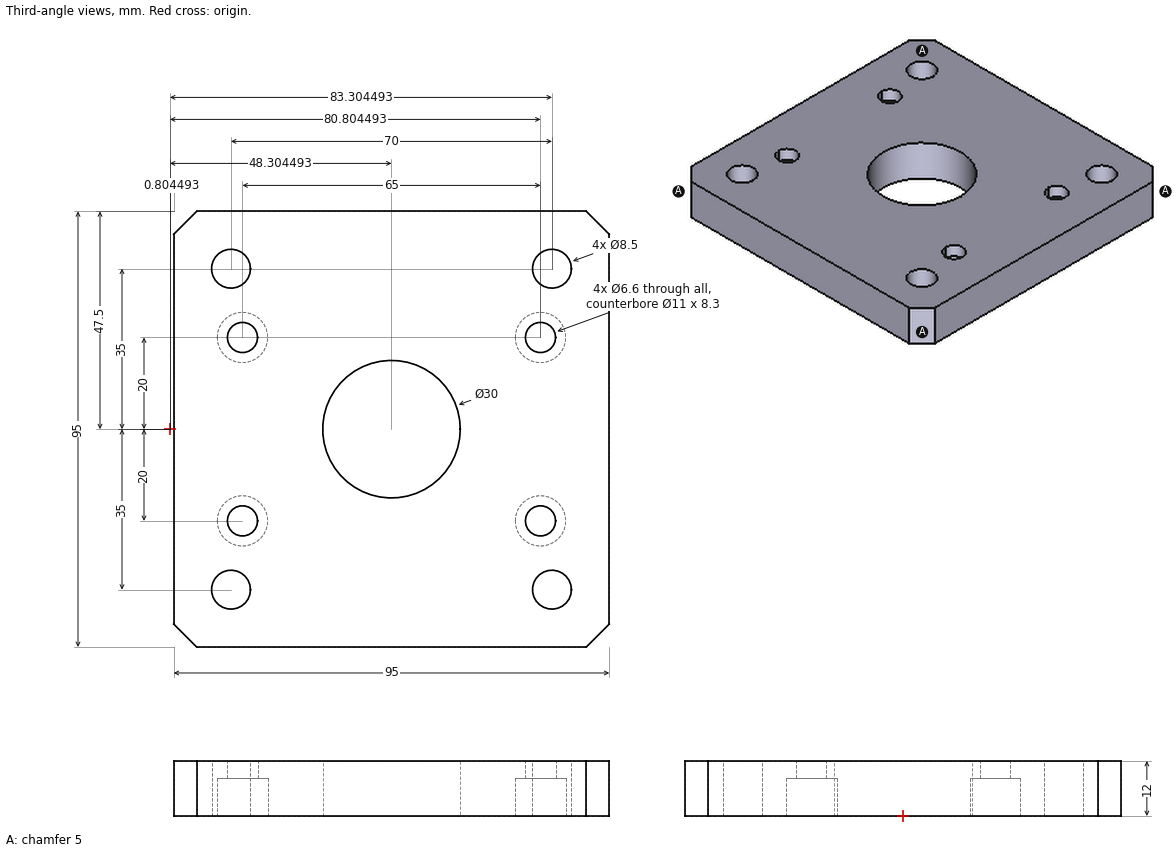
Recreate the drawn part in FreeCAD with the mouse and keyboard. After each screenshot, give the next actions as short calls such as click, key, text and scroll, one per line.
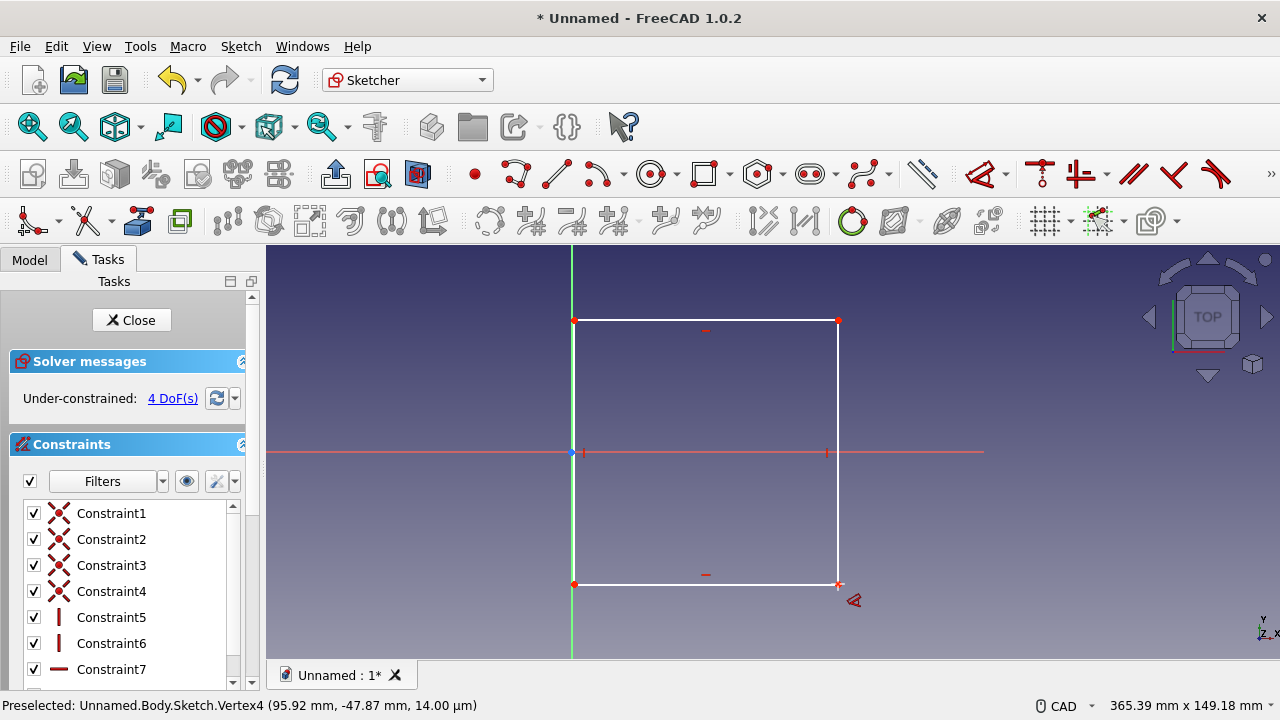
click(574, 400)
click(540, 392)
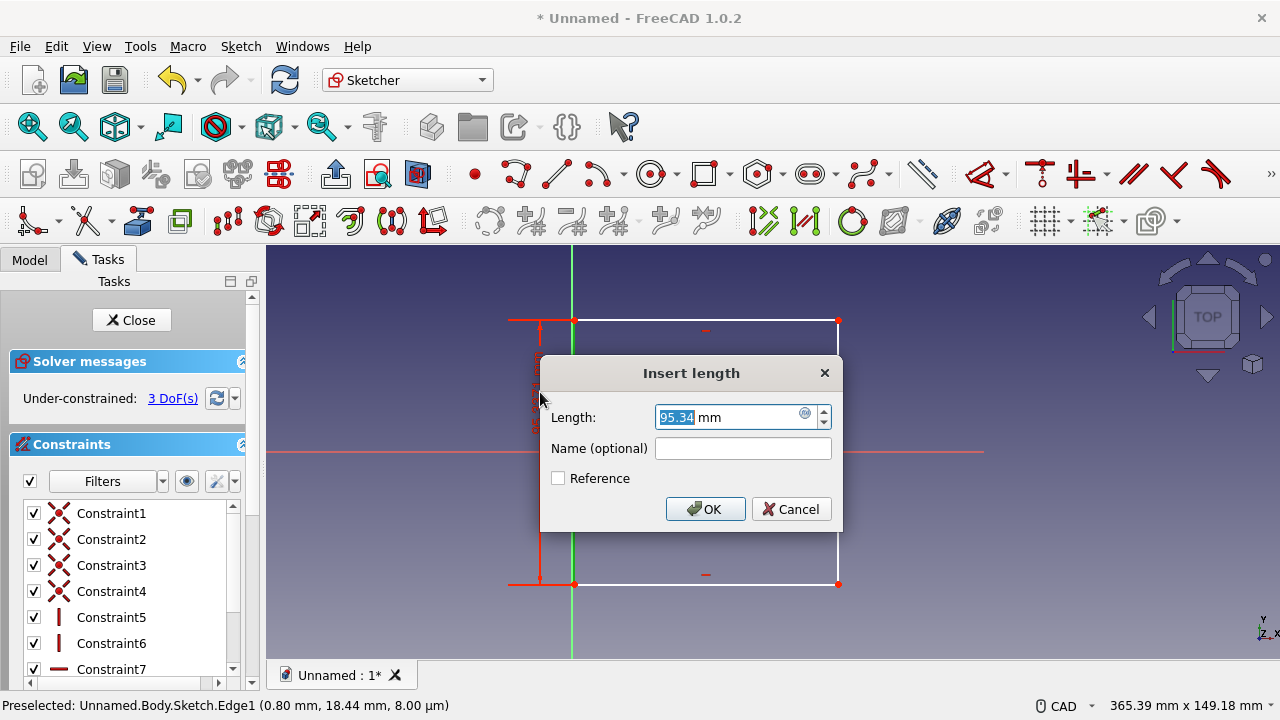
text(95)
key(Return)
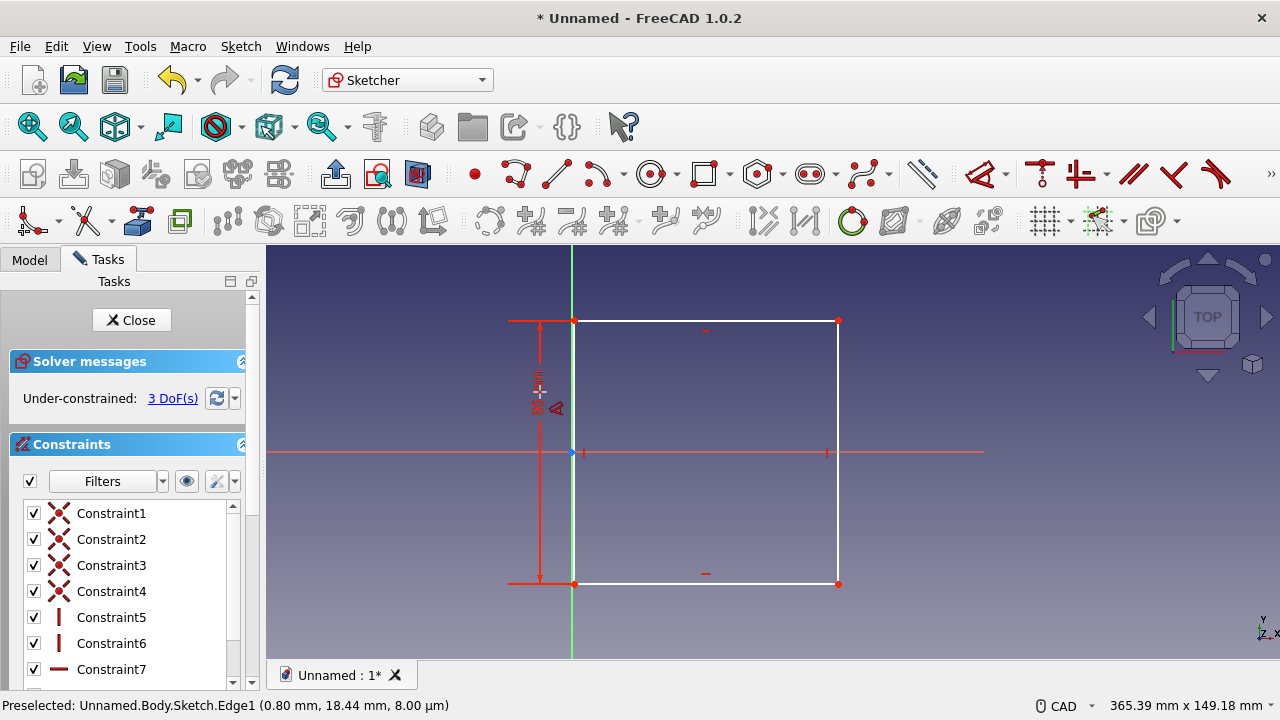
click(653, 584)
click(706, 618)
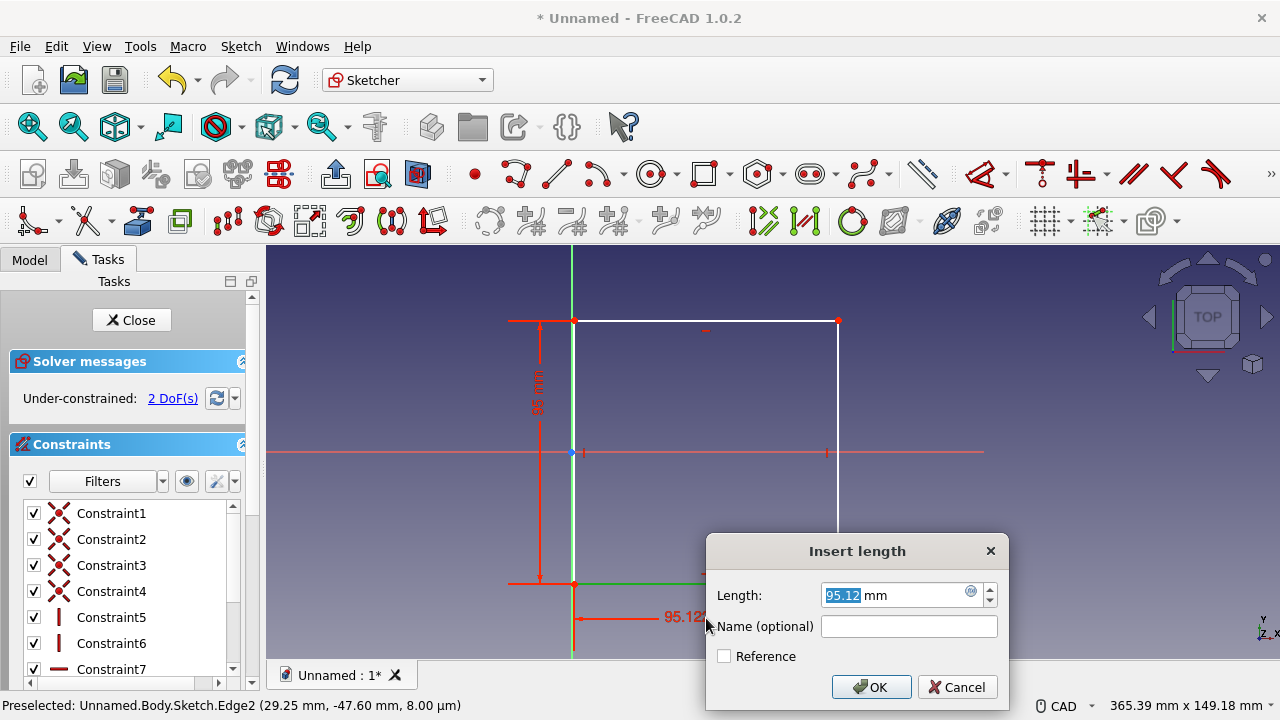
text(95)
key(Return)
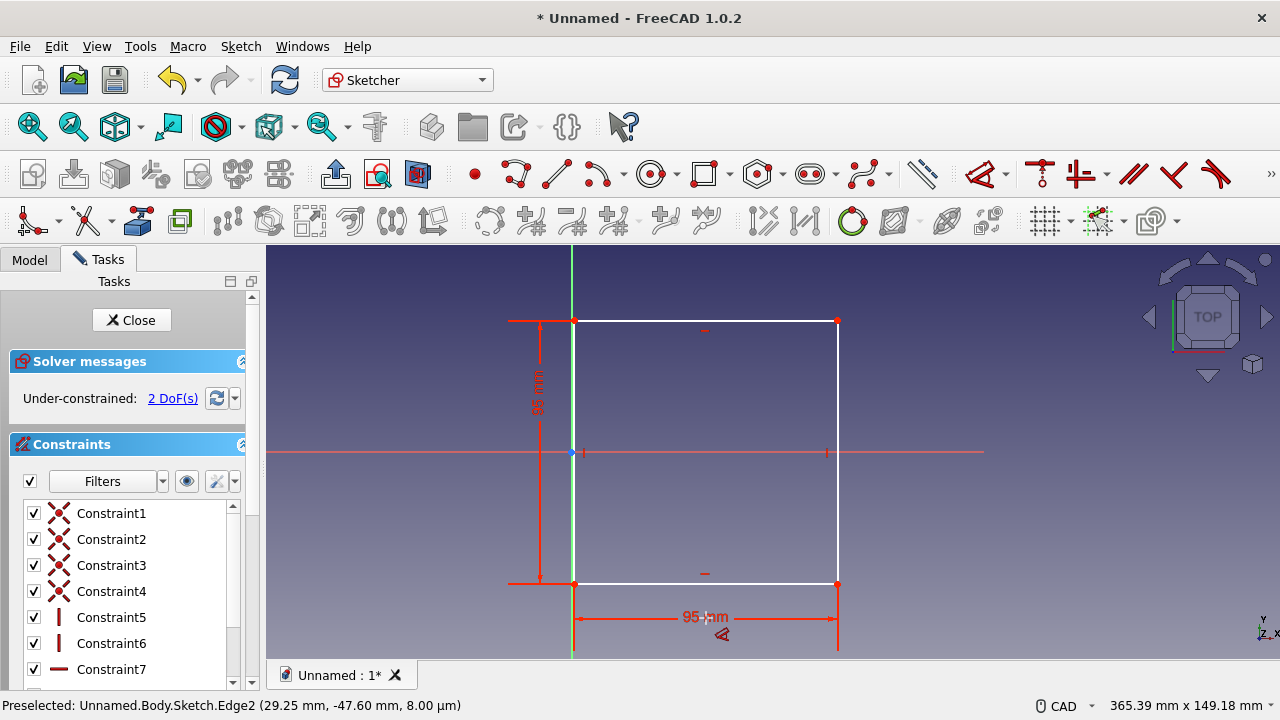
click(574, 321)
click(538, 356)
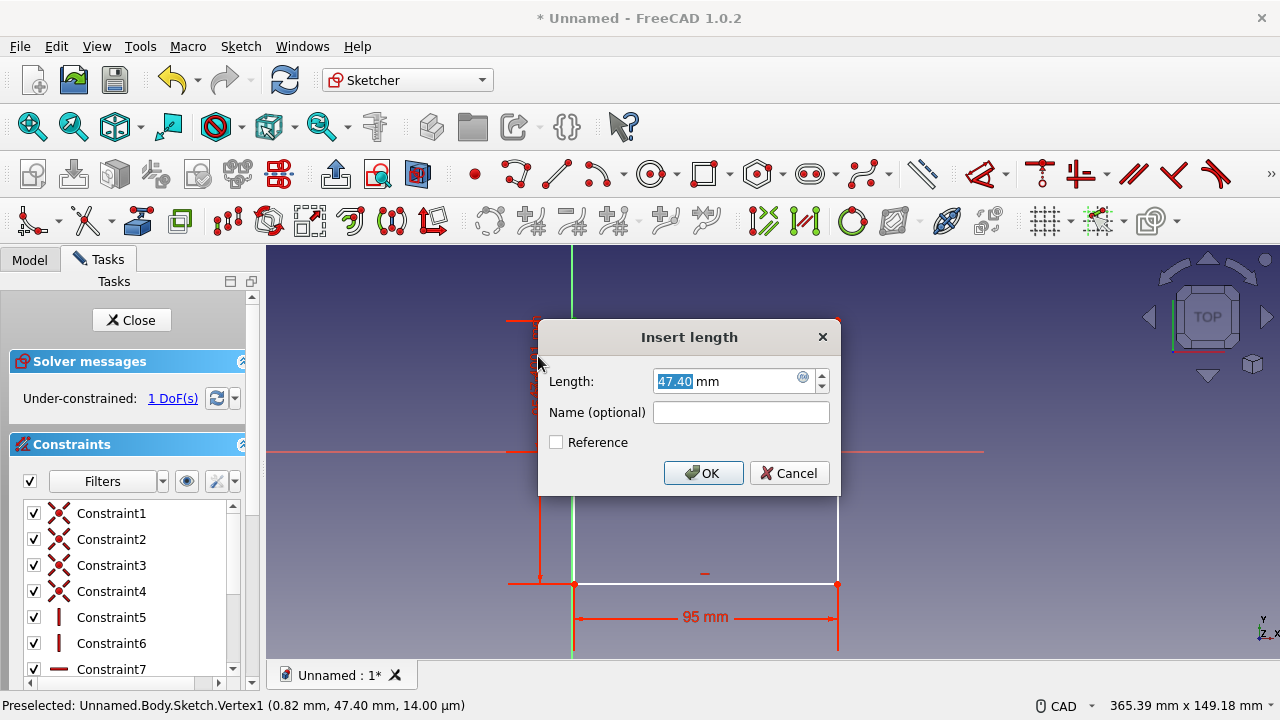
text(47.5)
key(Return)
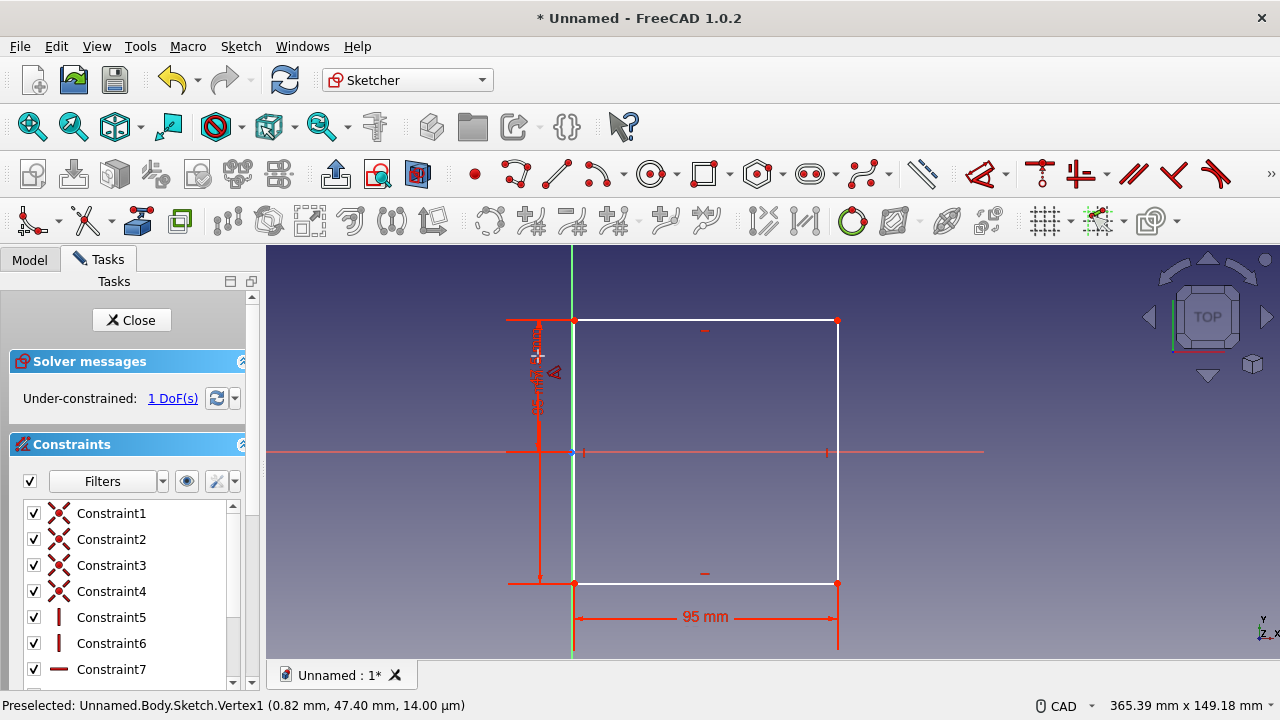
scroll(574, 320, up, 15)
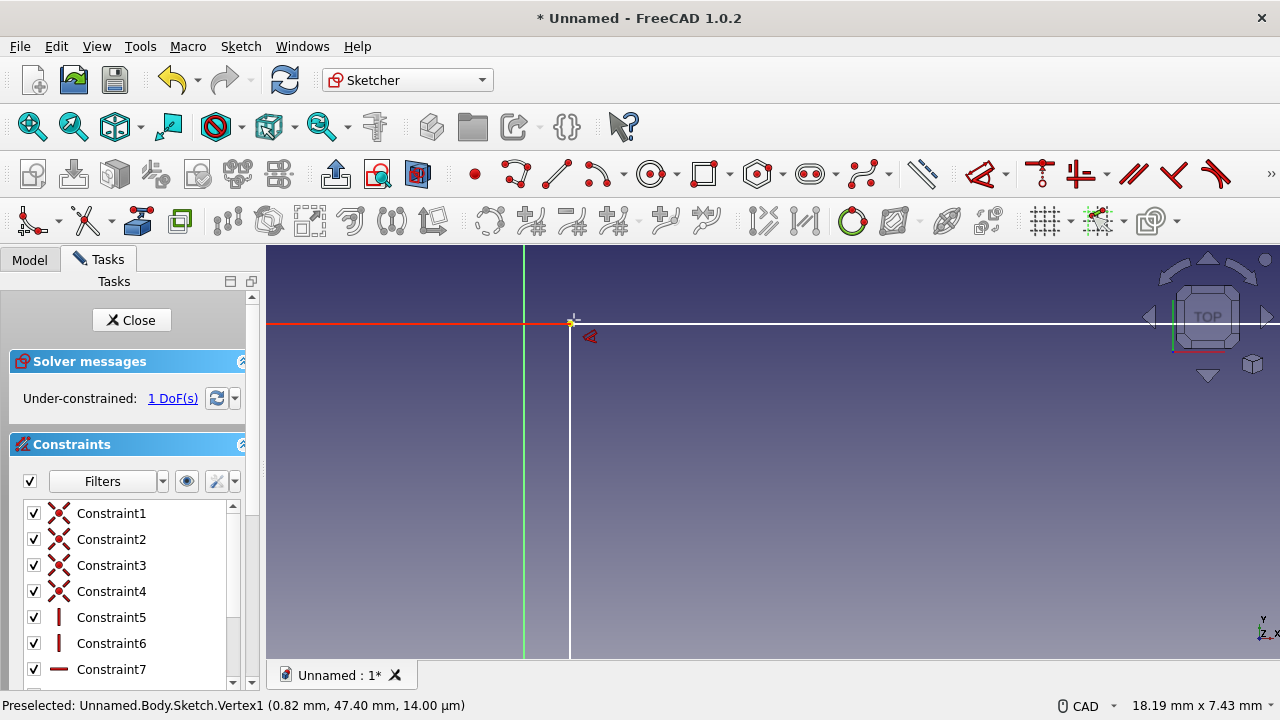
click(570, 324)
click(547, 290)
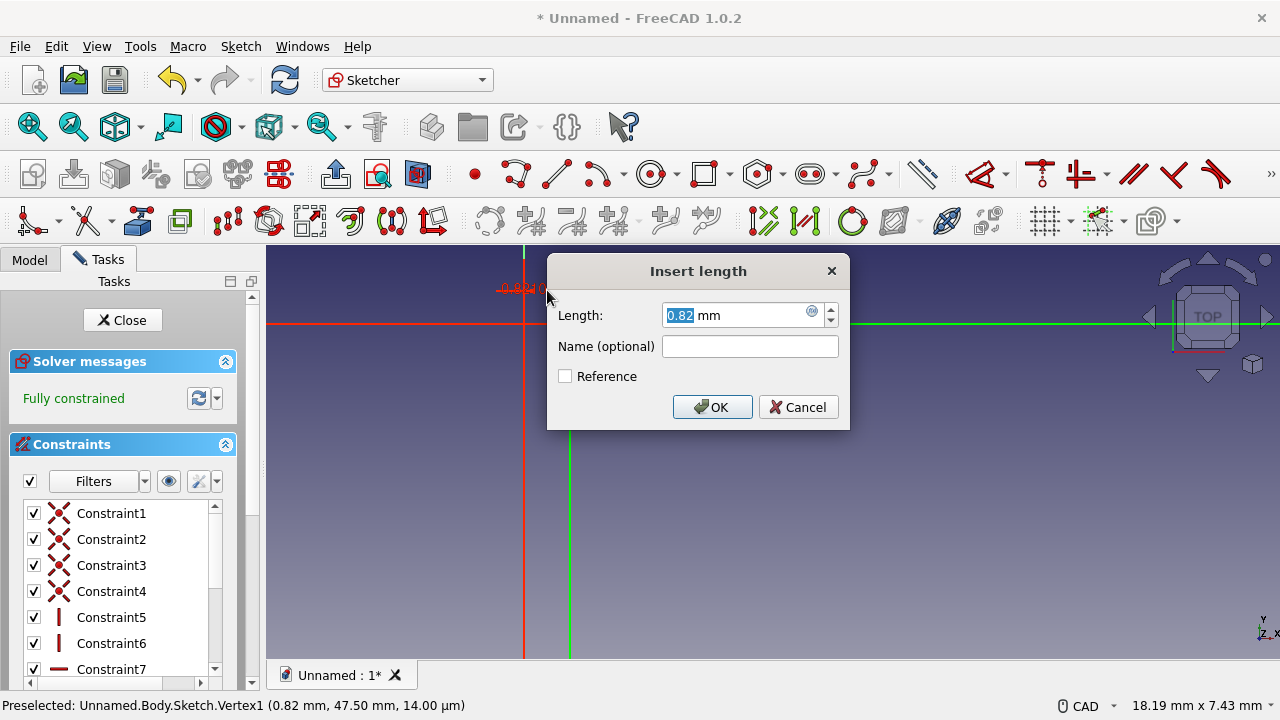
text(0.804493)
key(Return)
key(Escape)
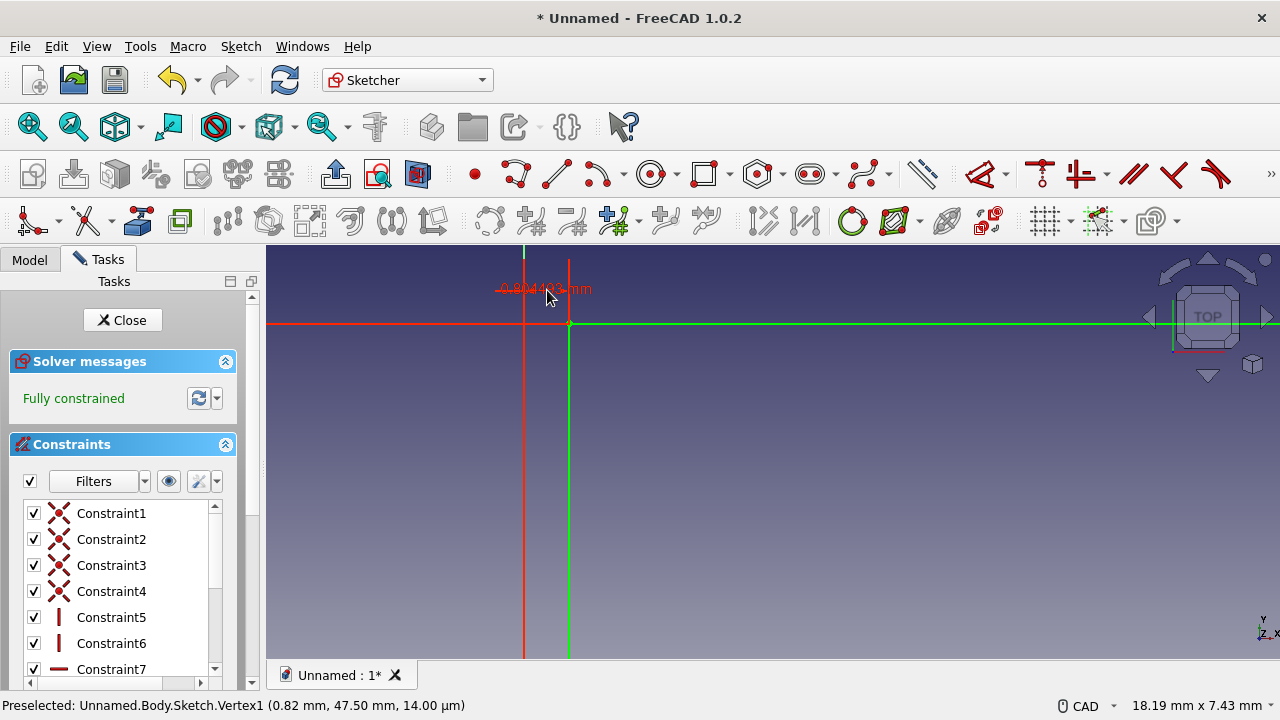
click(123, 320)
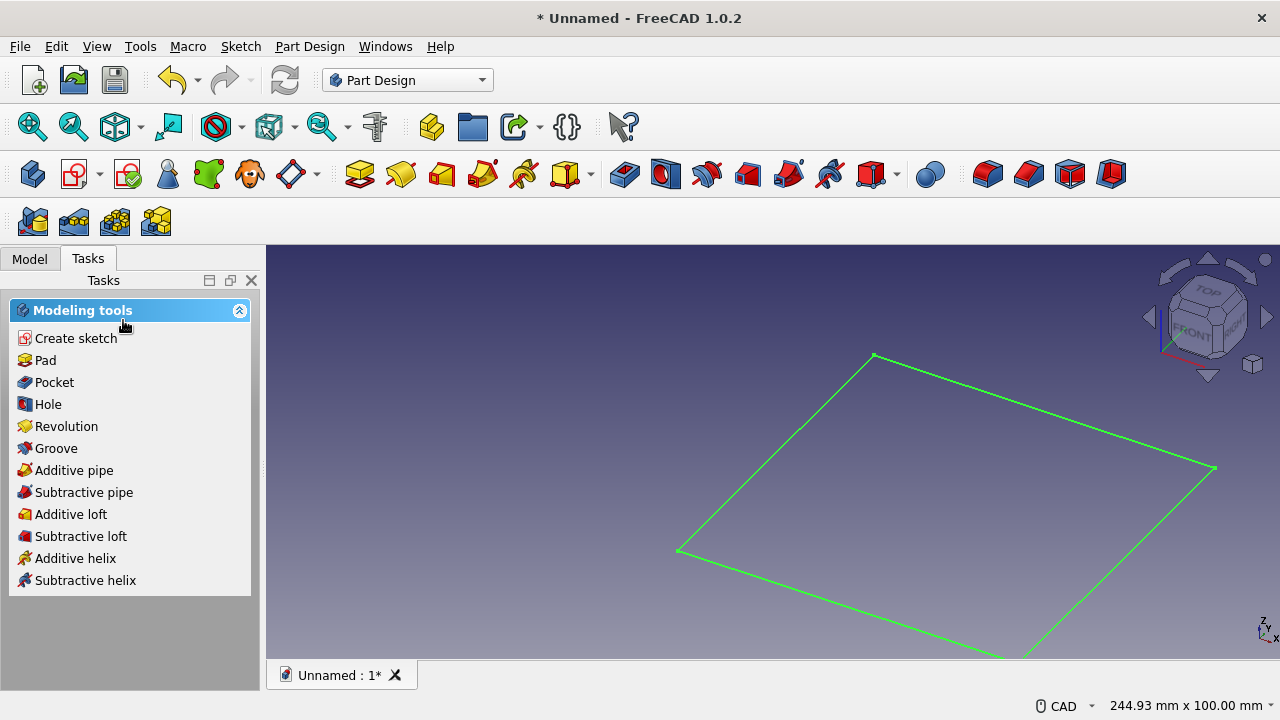
click(360, 174)